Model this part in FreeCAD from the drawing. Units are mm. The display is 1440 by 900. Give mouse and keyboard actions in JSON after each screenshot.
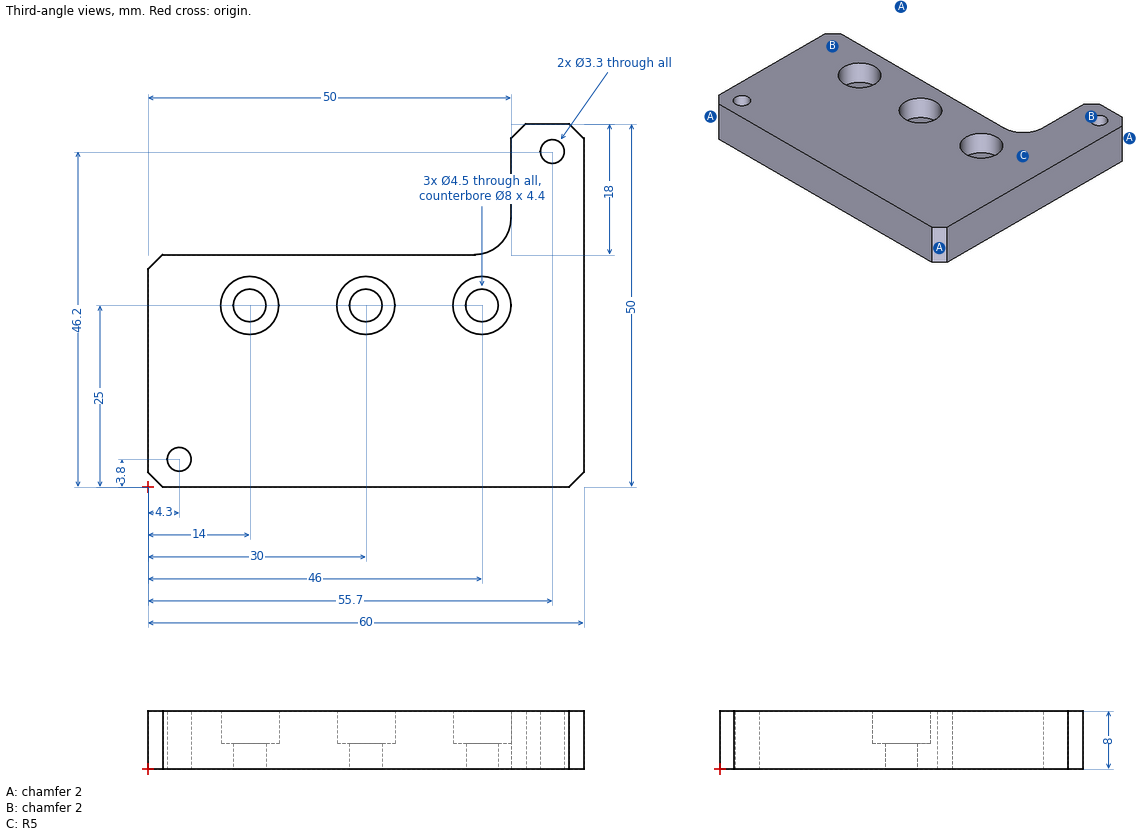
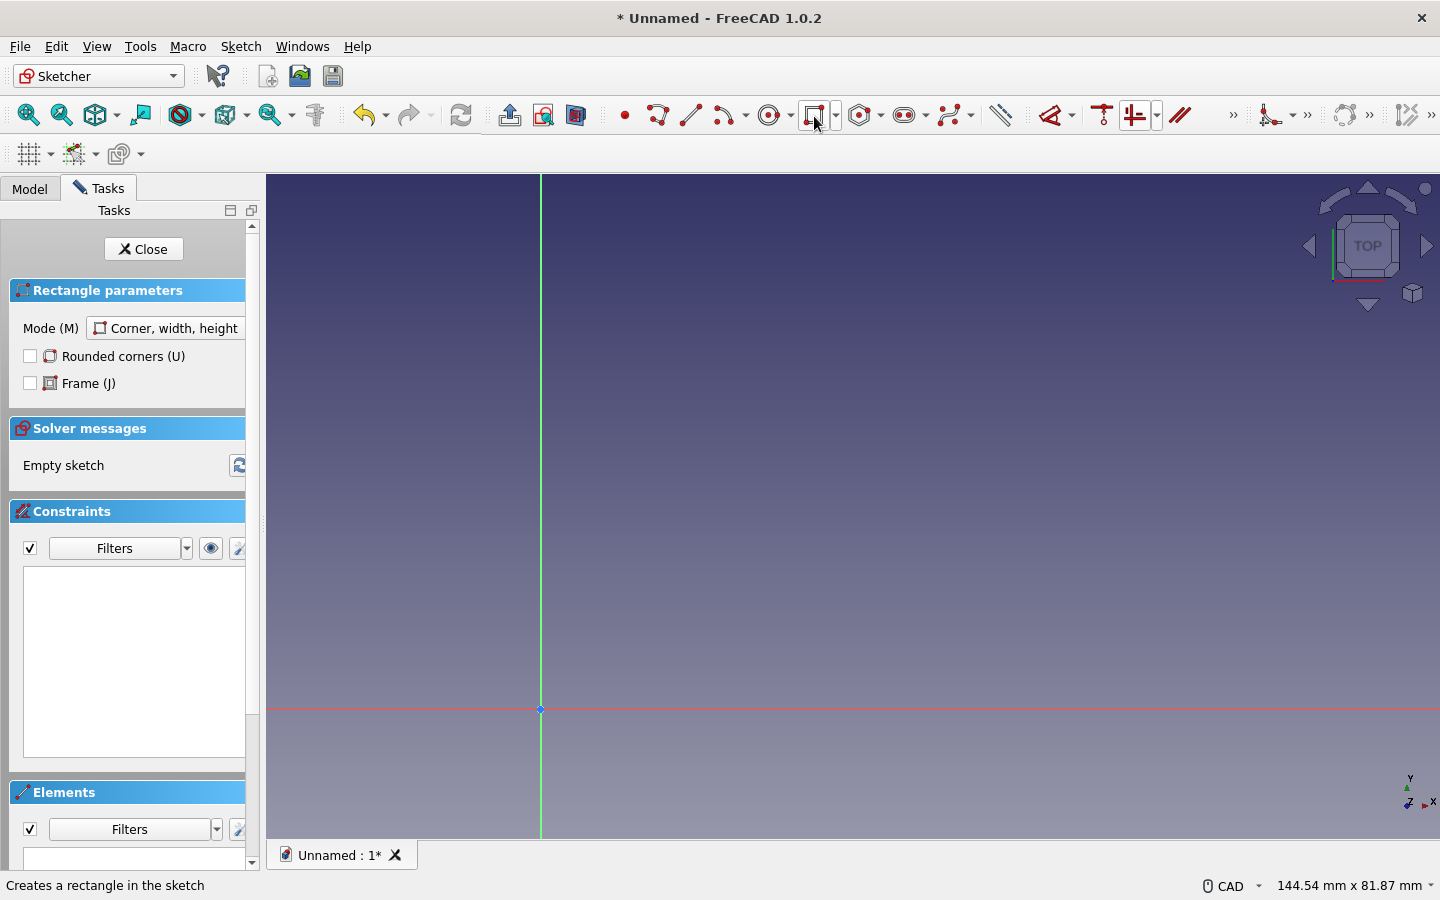
{"action": "left_click", "coordinate": [541, 709]}
{"action": "mouse_move", "coordinate": [1028, 303]}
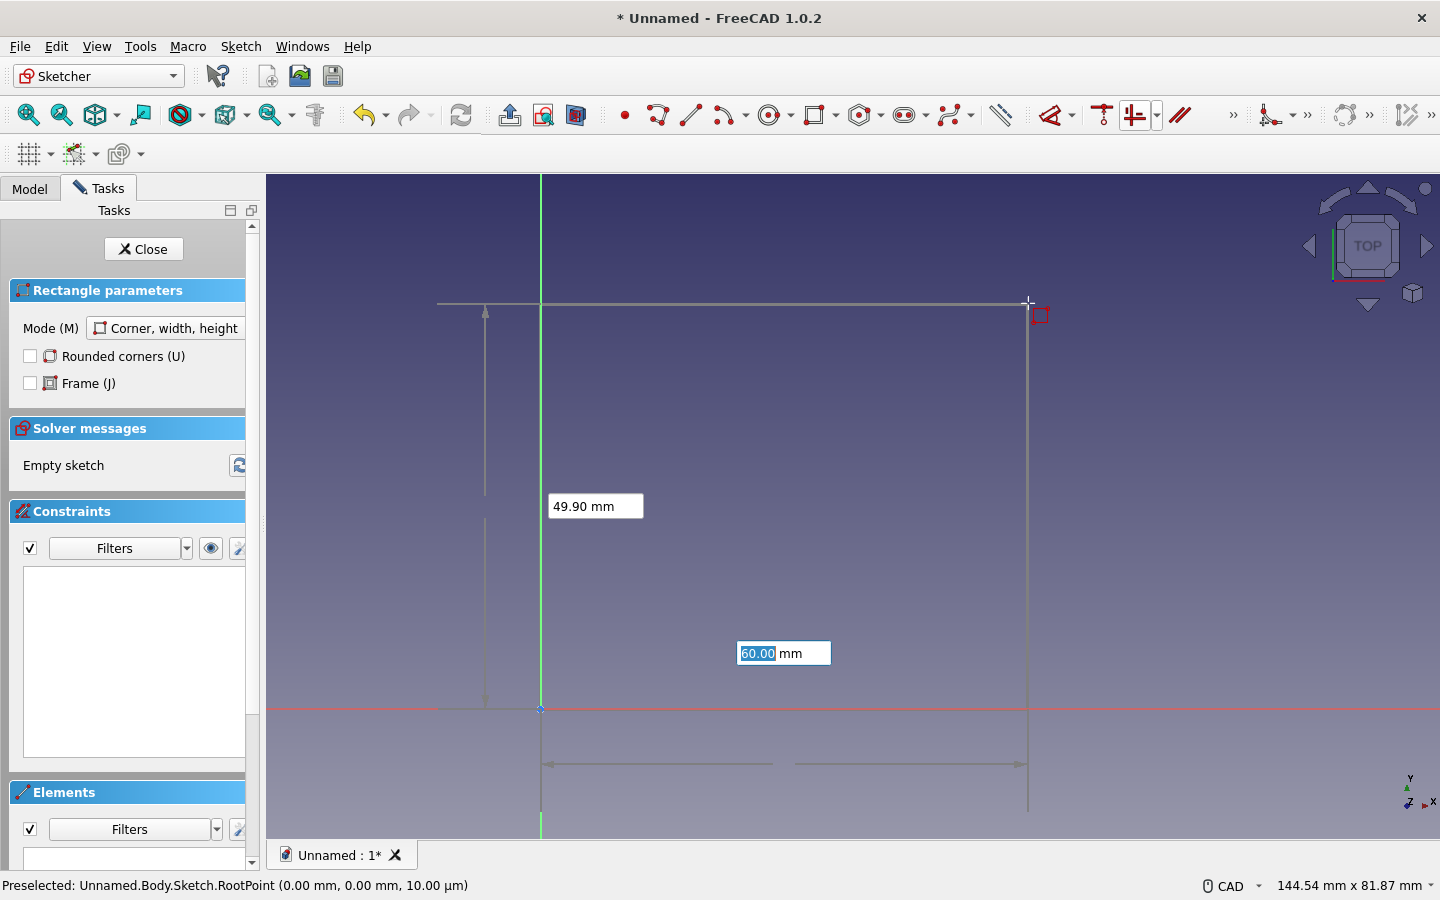
{"action": "type", "text": "60"}
{"action": "key", "text": "Tab"}
{"action": "type", "text": "50"}
{"action": "key", "text": "Return"}
{"action": "key", "text": "Escape"}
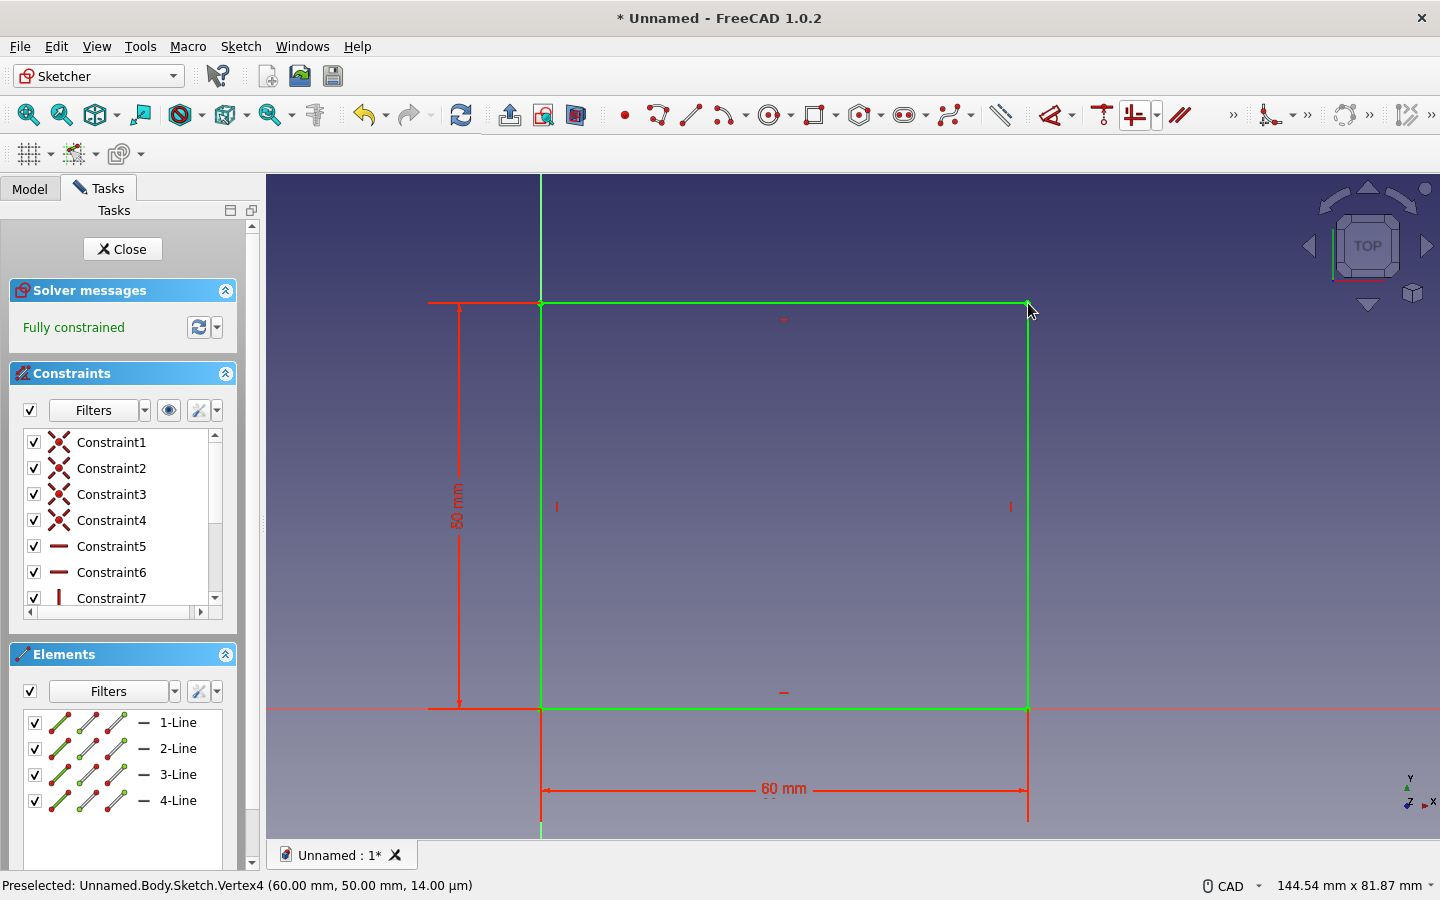
{"action": "left_click", "coordinate": [123, 249]}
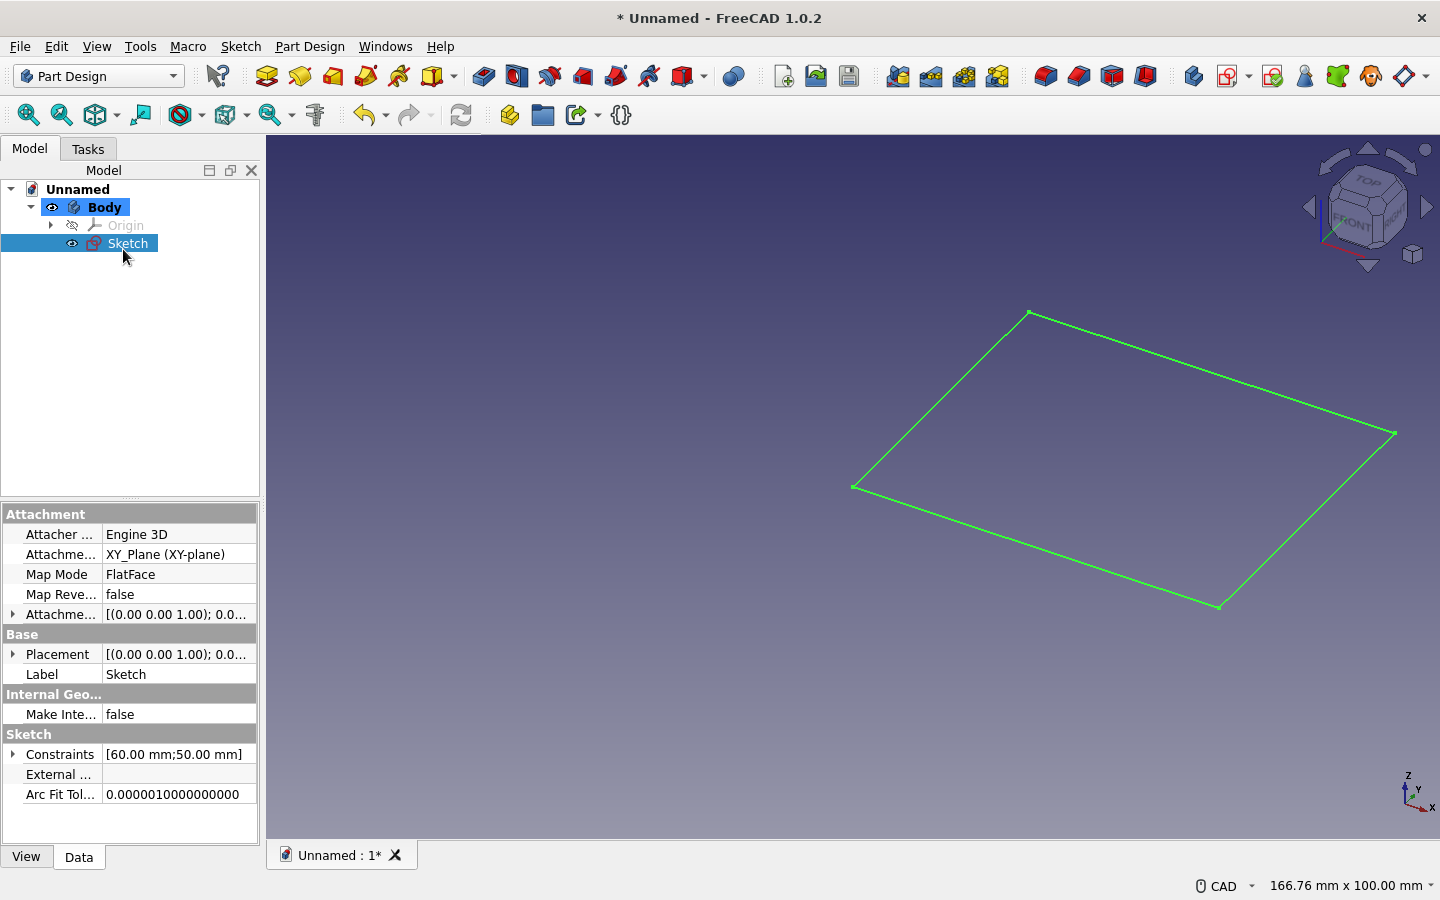
{"action": "left_click", "coordinate": [267, 76]}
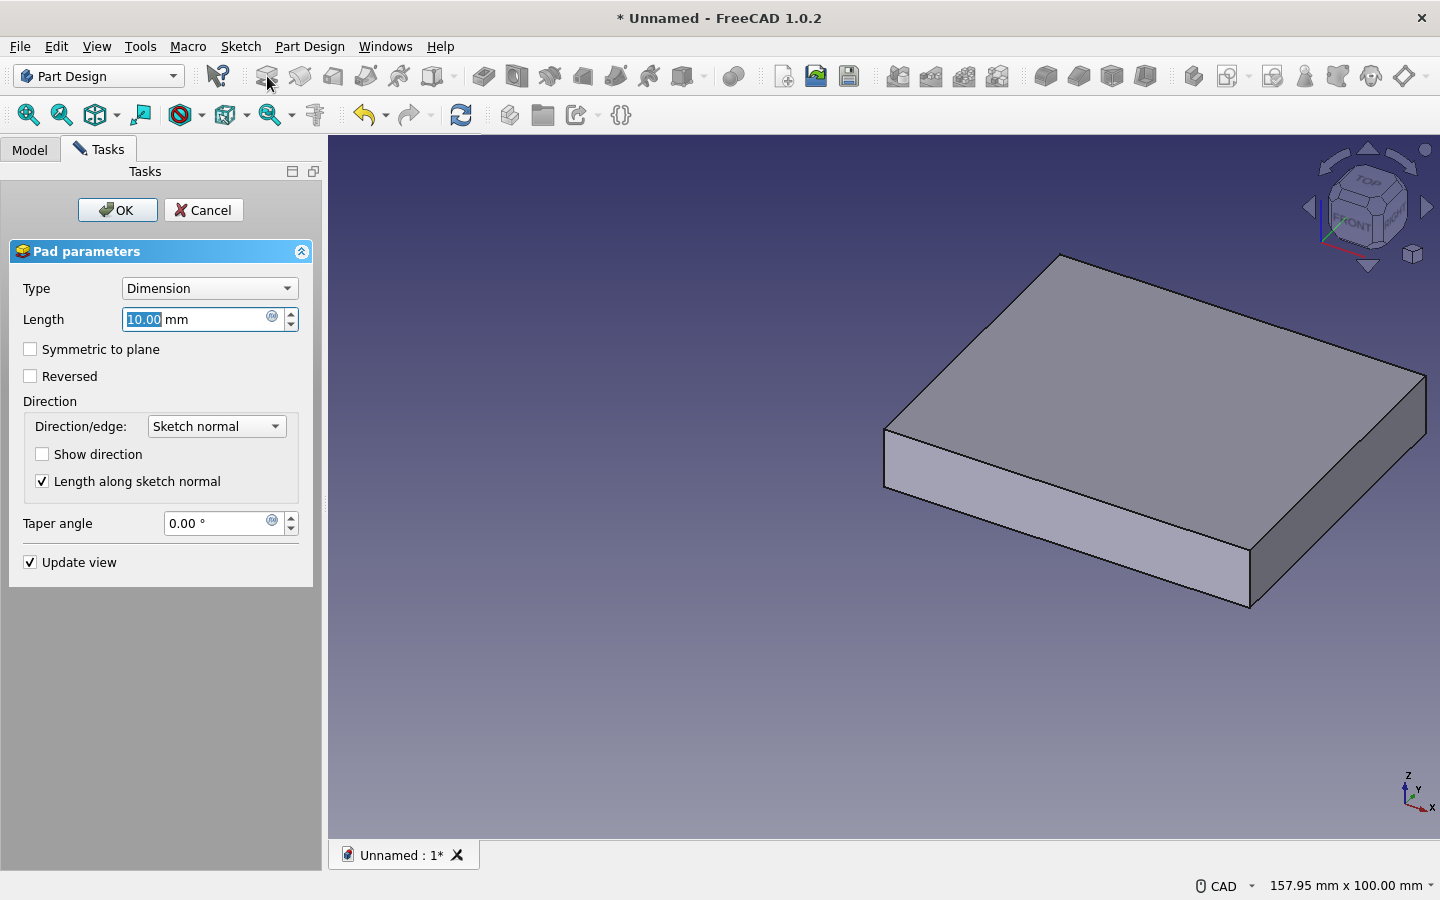
{"action": "type", "text": "8"}
{"action": "key", "text": "Tab"}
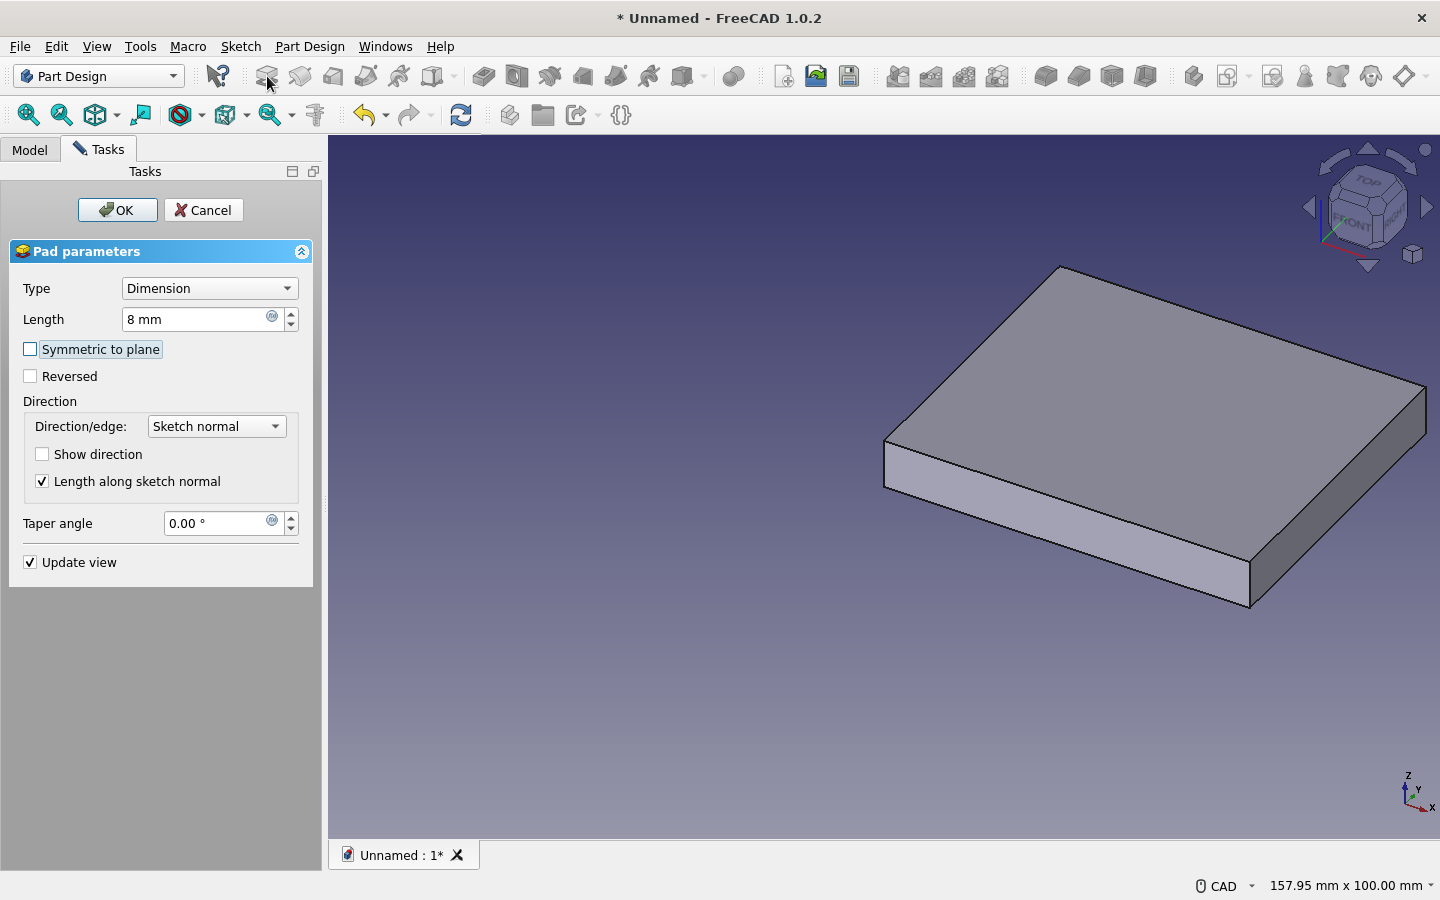
{"action": "left_click", "coordinate": [118, 210]}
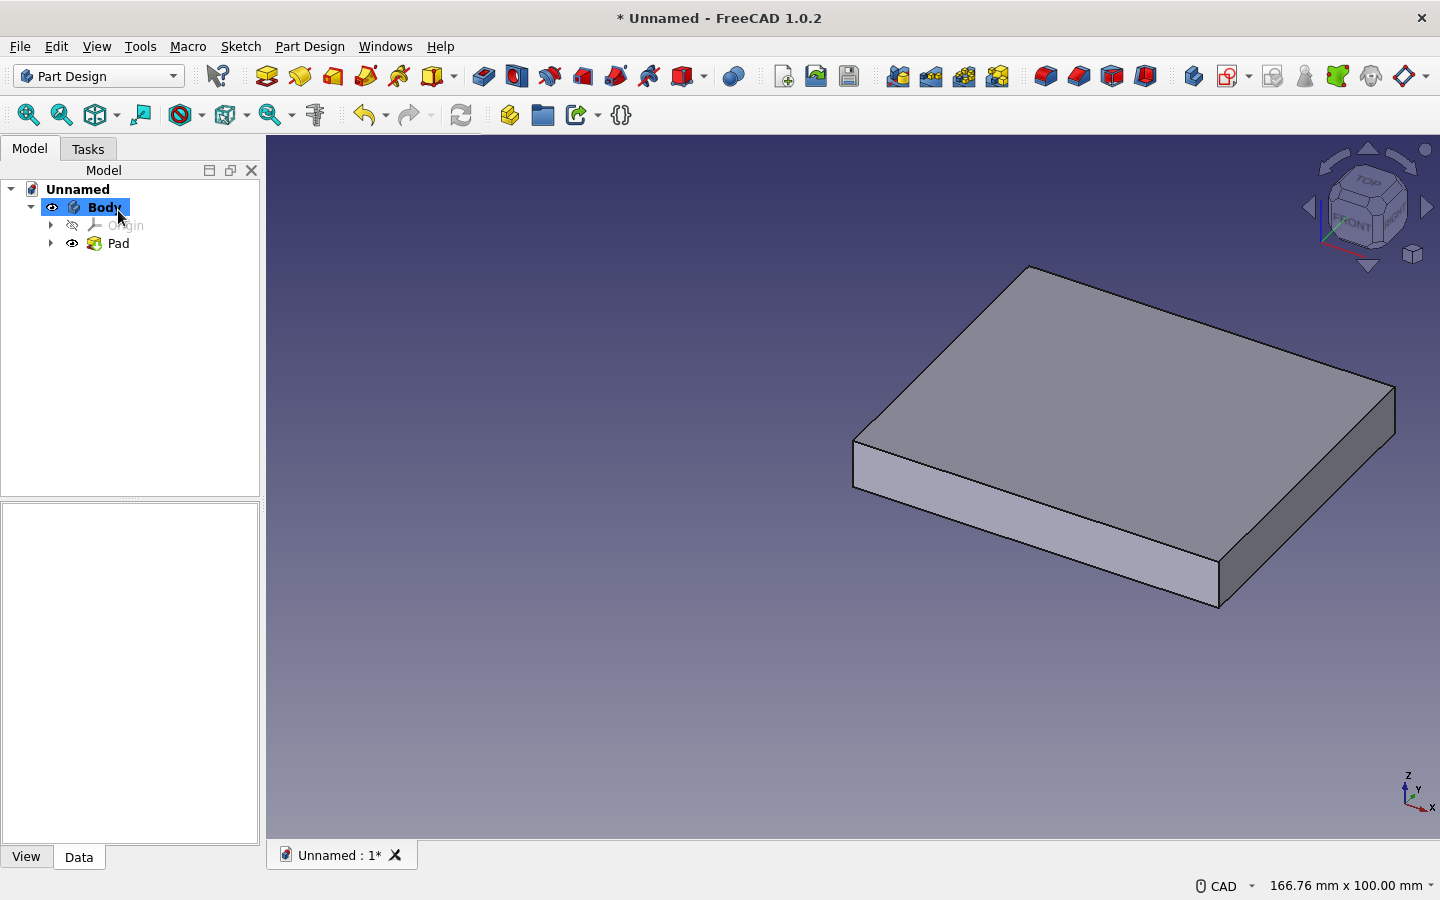
{"action": "left_click", "coordinate": [1124, 413]}